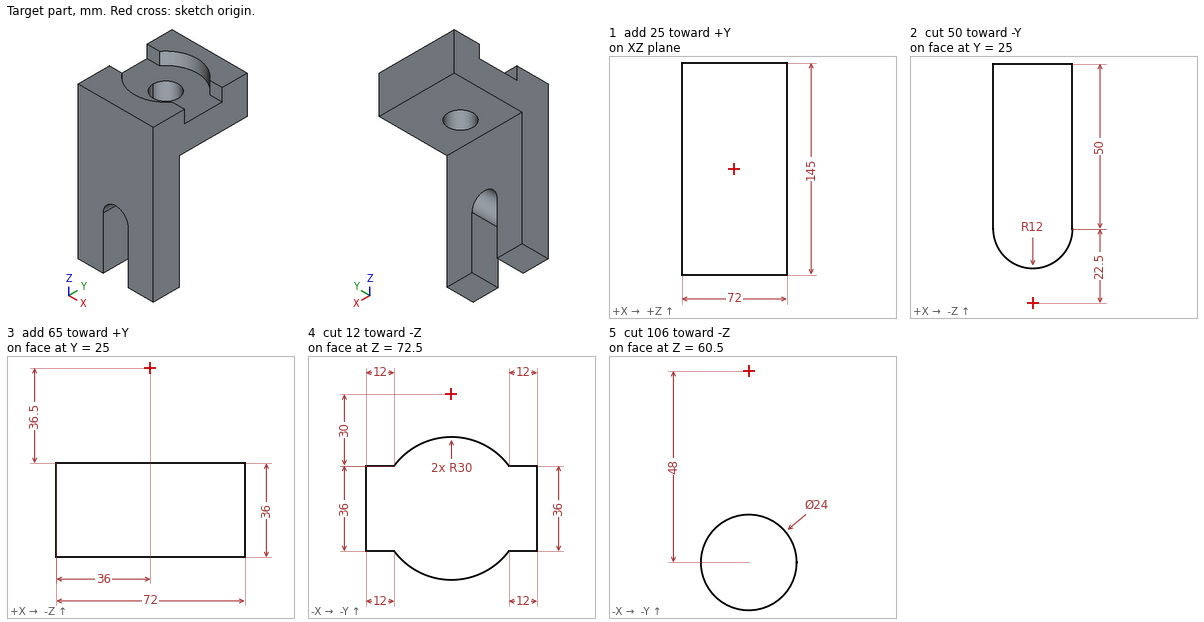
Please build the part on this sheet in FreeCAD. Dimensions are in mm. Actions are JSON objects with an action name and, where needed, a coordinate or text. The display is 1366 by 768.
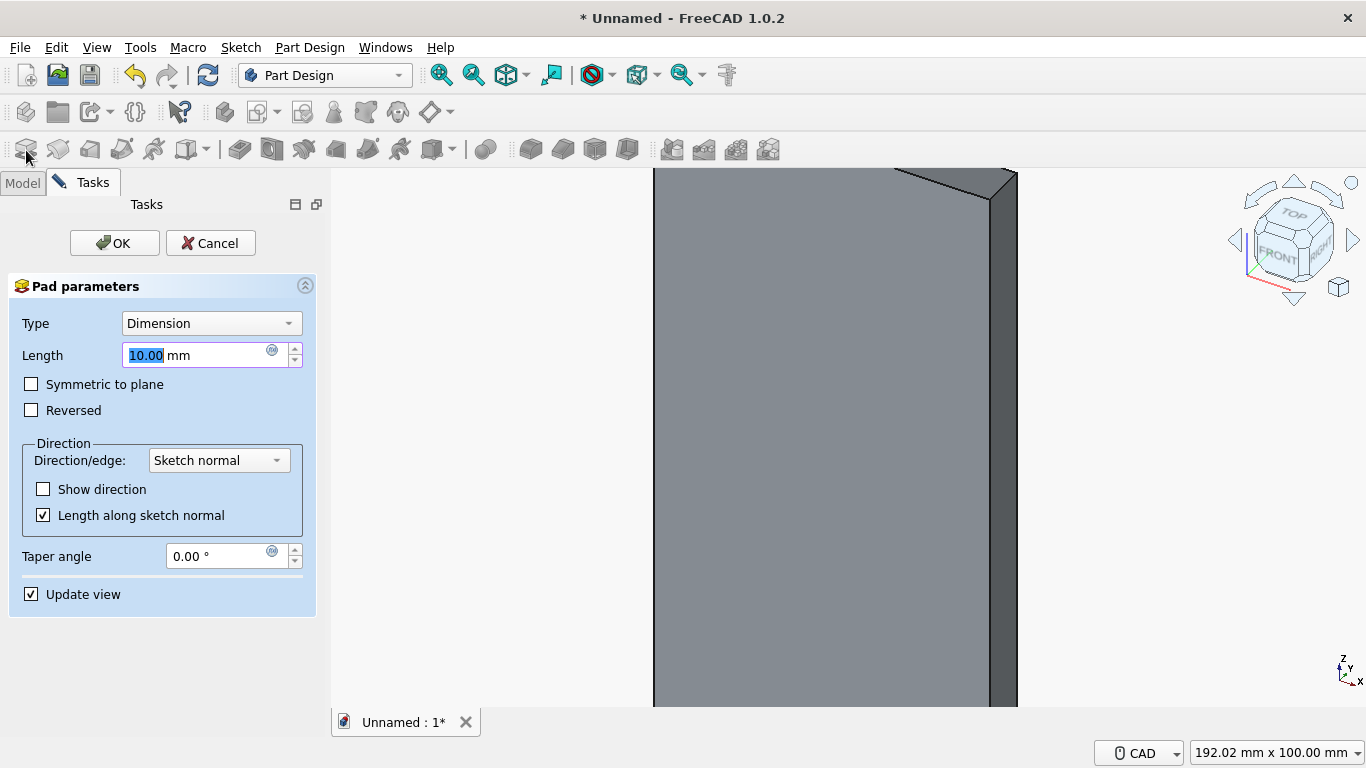
{"action": "type", "text": "25"}
{"action": "key", "text": "Tab"}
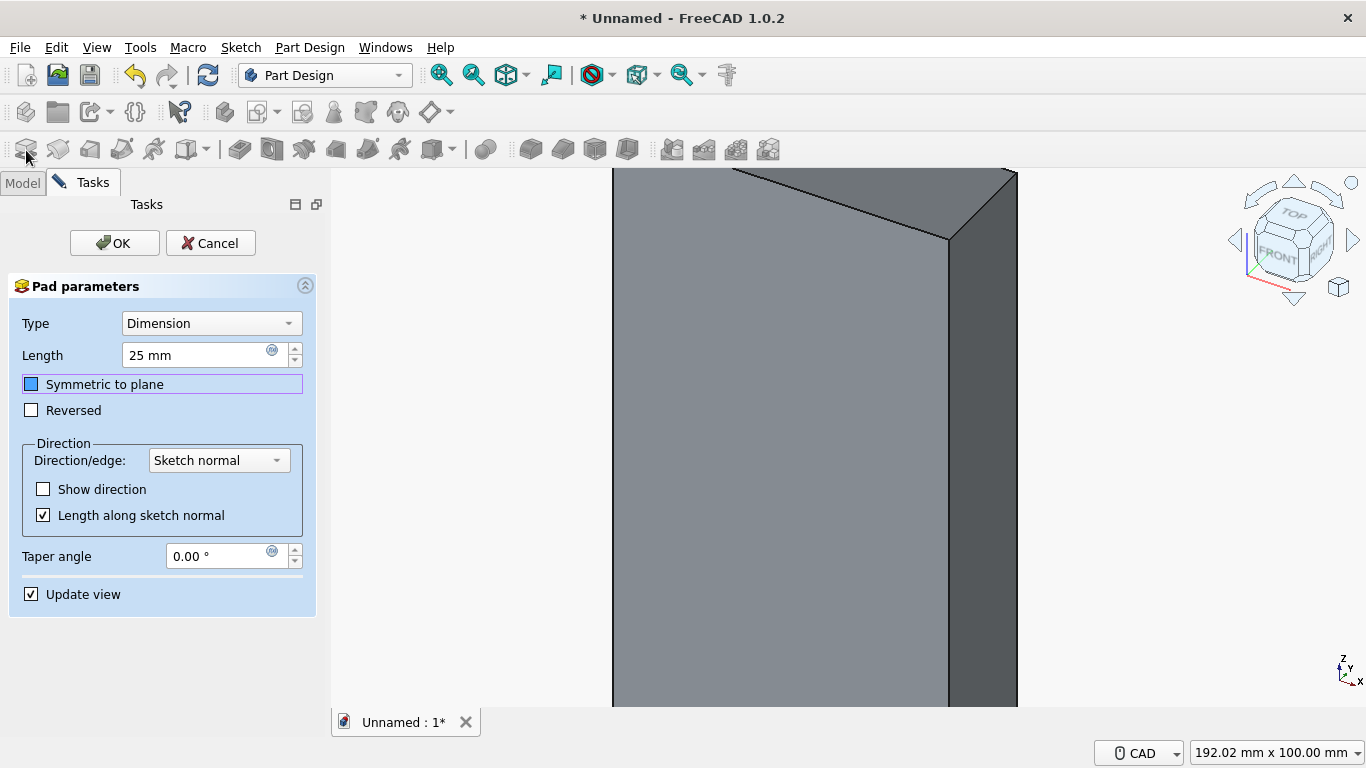
{"action": "left_click", "coordinate": [30, 410]}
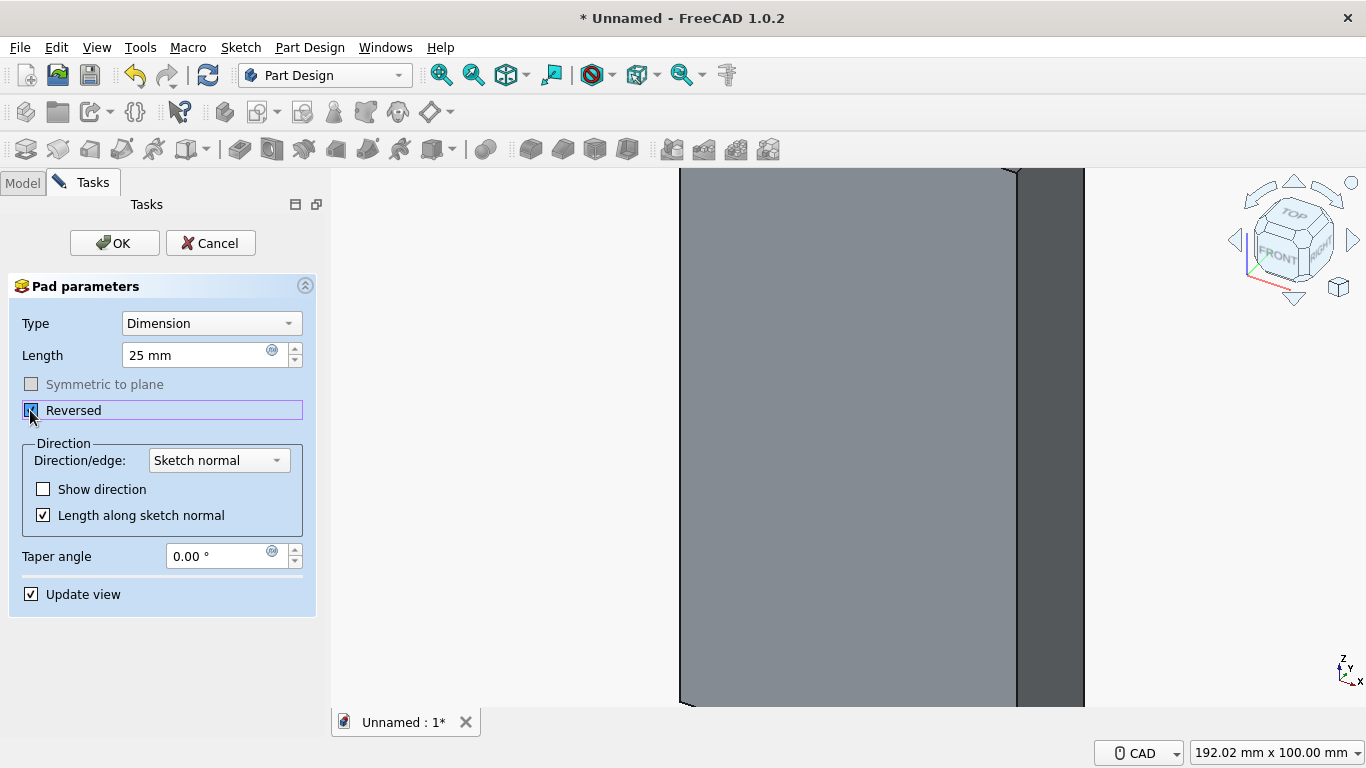
{"action": "left_click", "coordinate": [115, 243]}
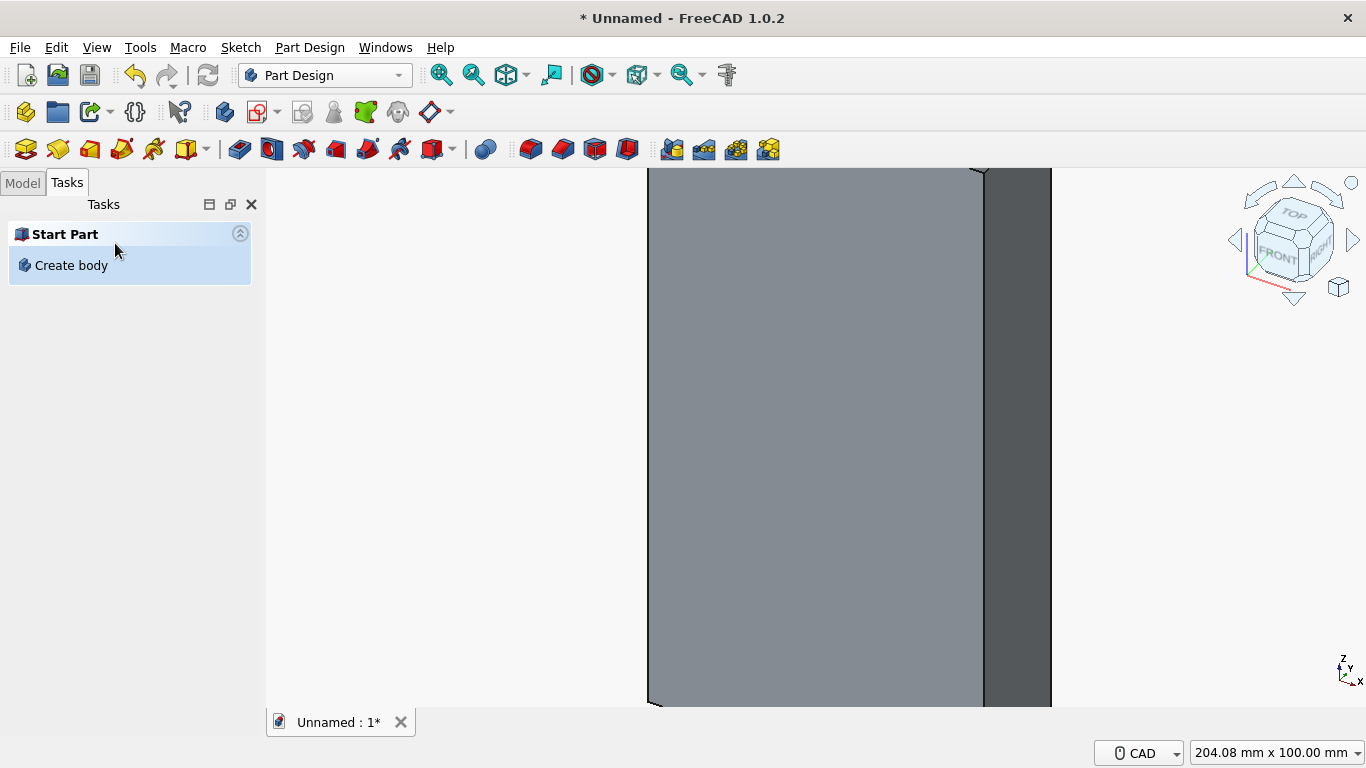
{"action": "left_click", "coordinate": [442, 76]}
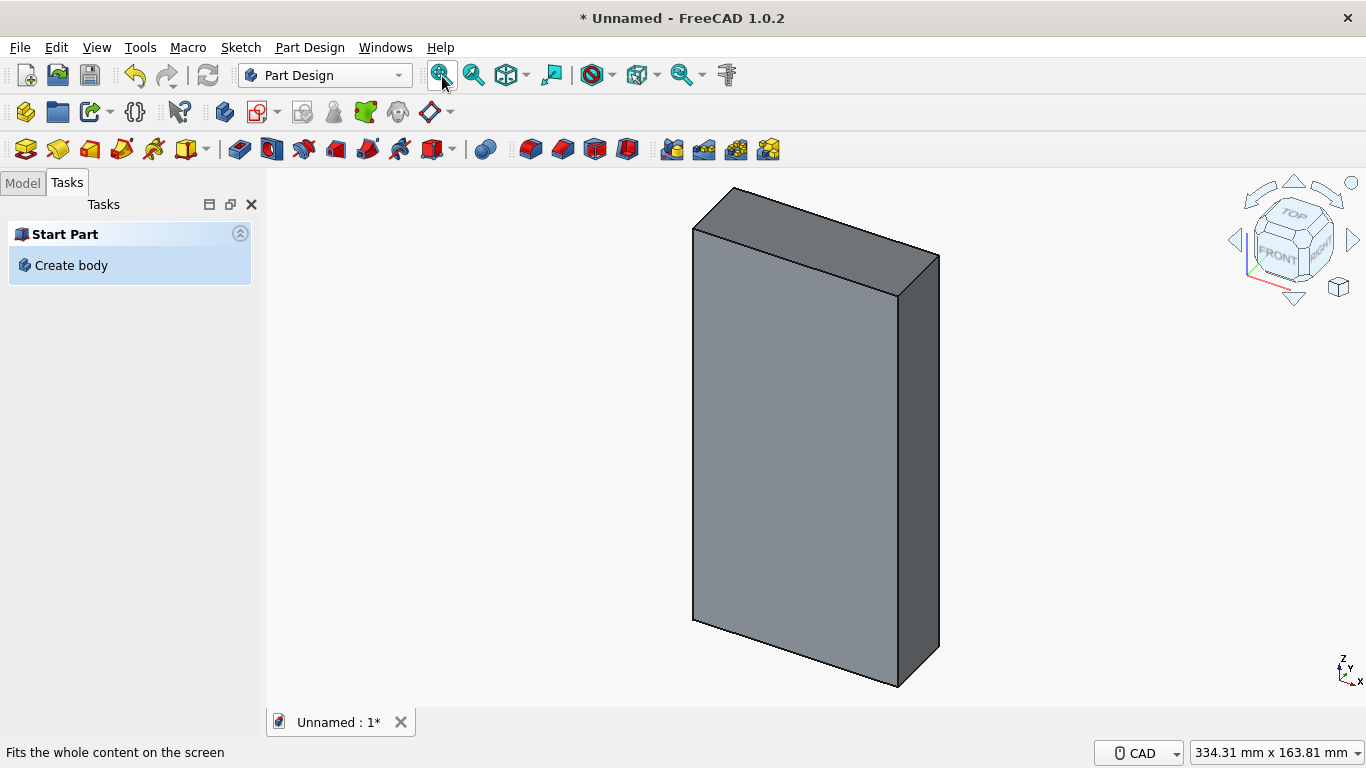
{"action": "key", "text": "4"}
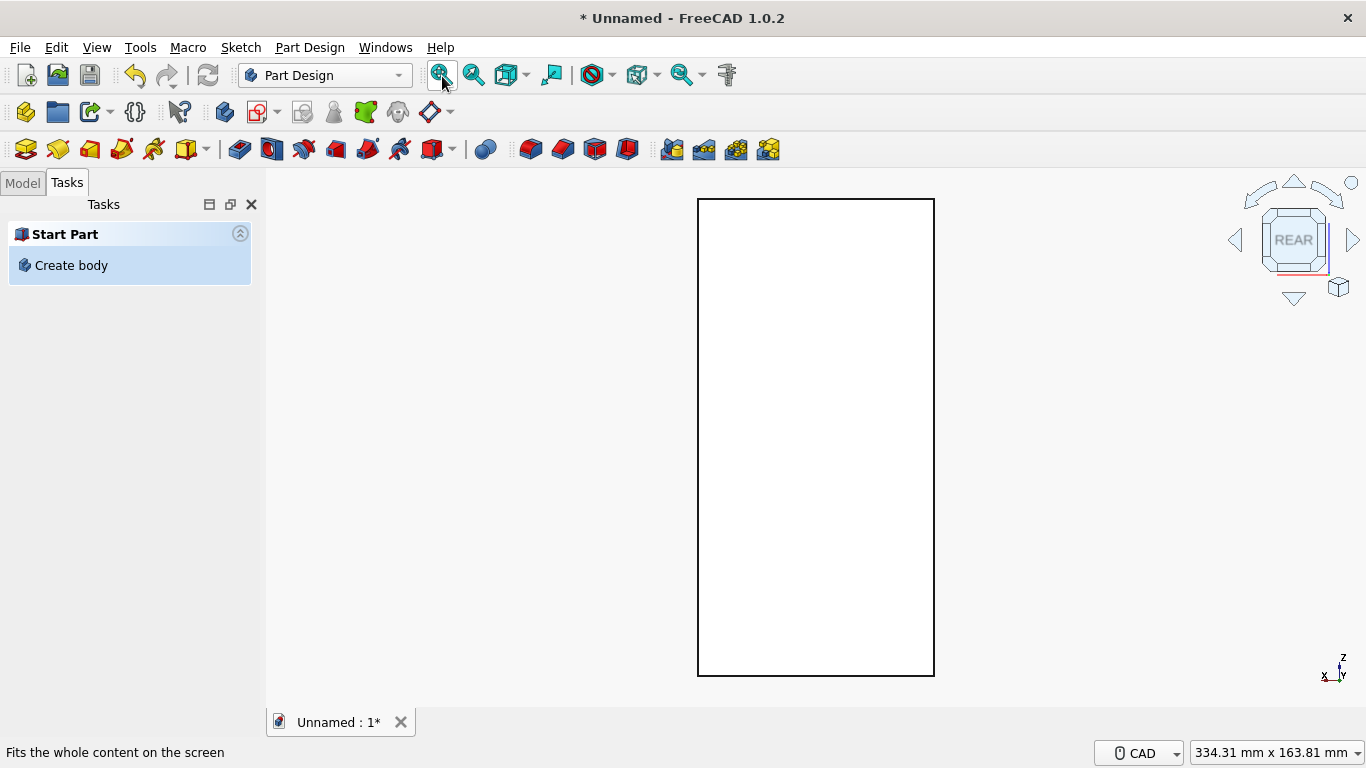
{"action": "left_click", "coordinate": [816, 368]}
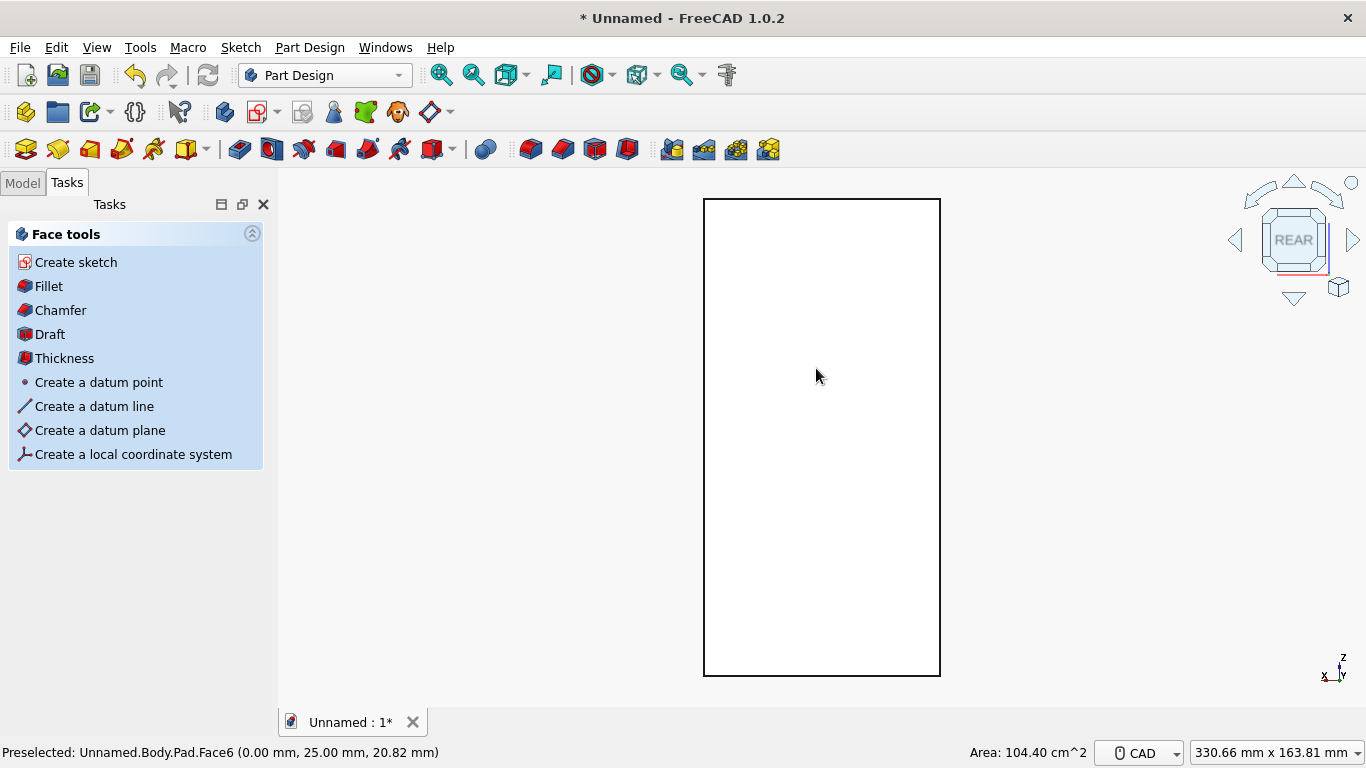
{"action": "left_click", "coordinate": [258, 112]}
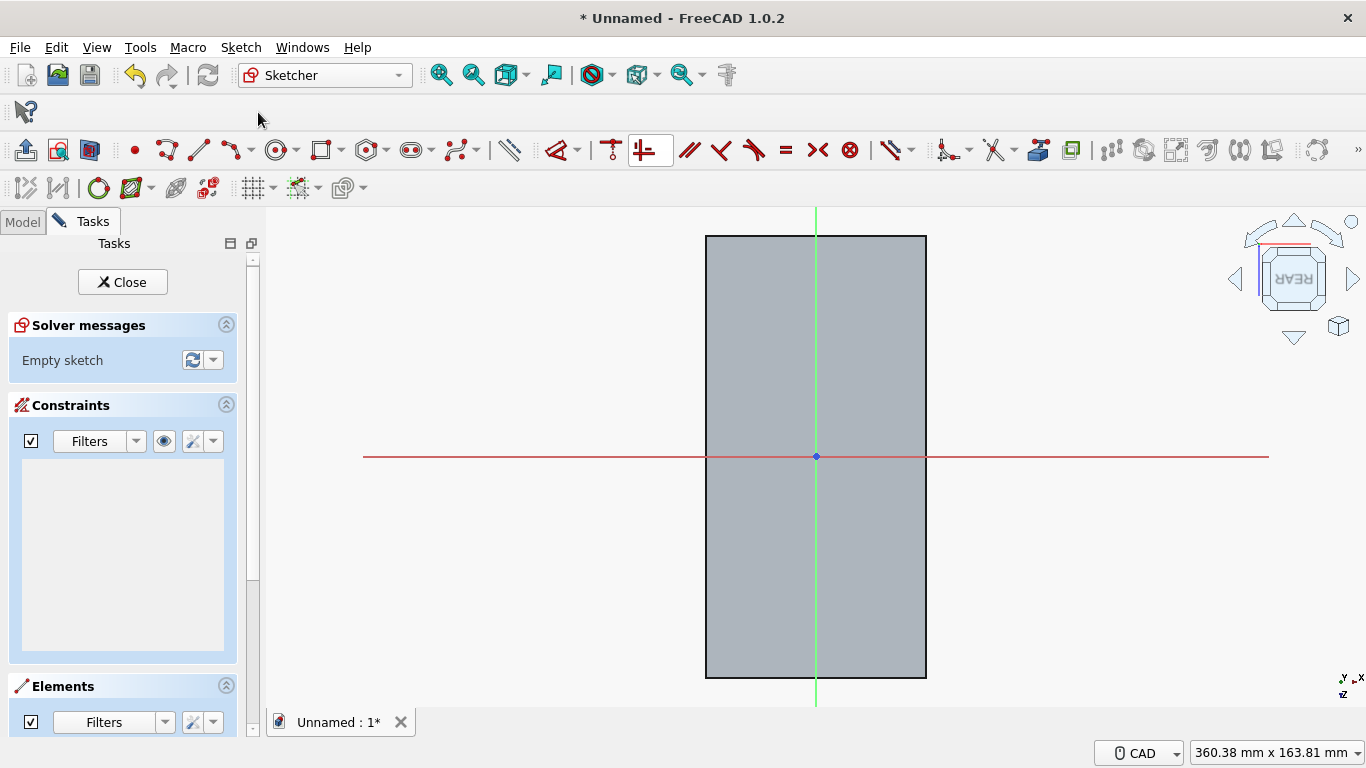
{"action": "scroll", "coordinate": [438, 679], "scroll_direction": "down", "scroll_amount": 1}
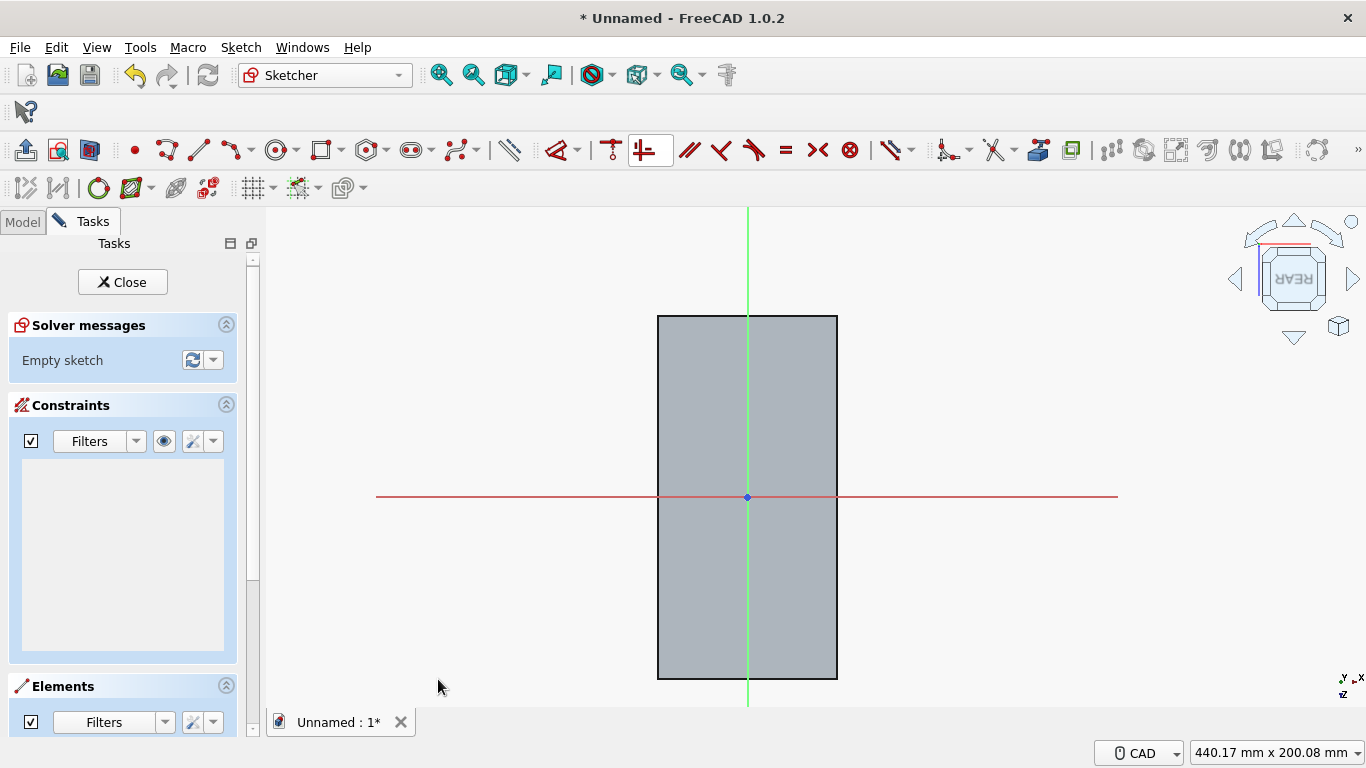
{"action": "scroll", "coordinate": [748, 346], "scroll_direction": "up", "scroll_amount": 3}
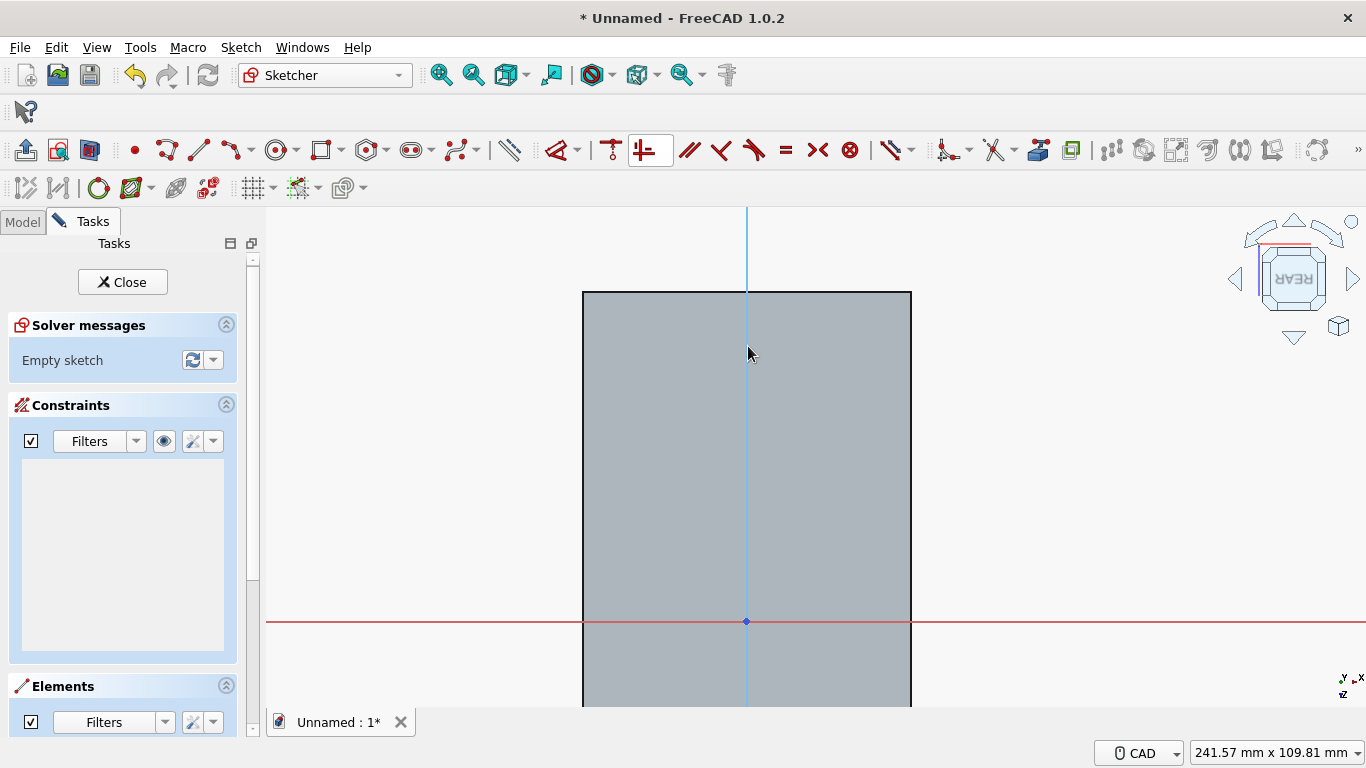
{"action": "left_click", "coordinate": [168, 150]}